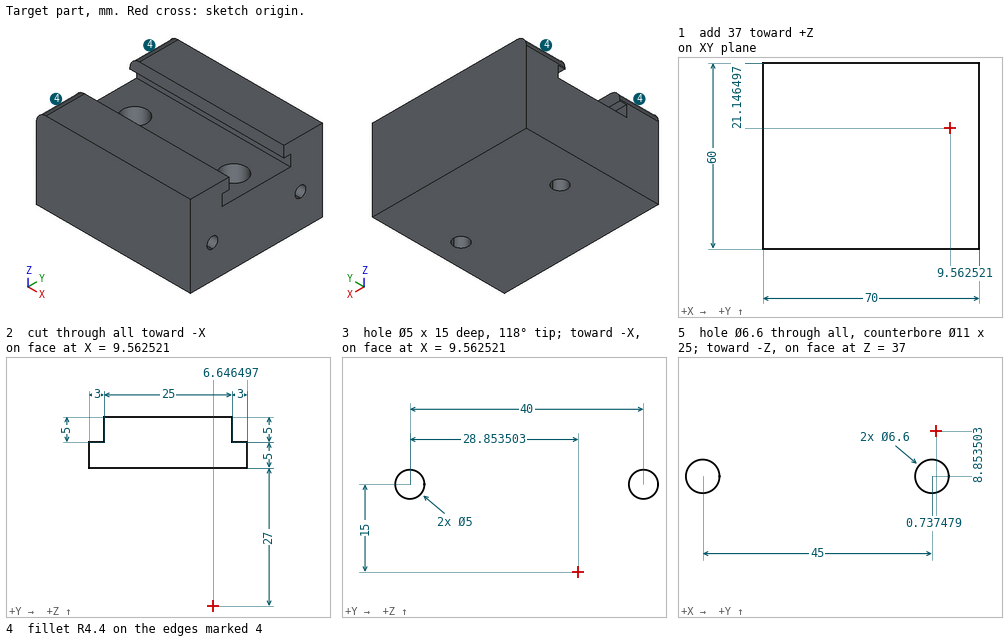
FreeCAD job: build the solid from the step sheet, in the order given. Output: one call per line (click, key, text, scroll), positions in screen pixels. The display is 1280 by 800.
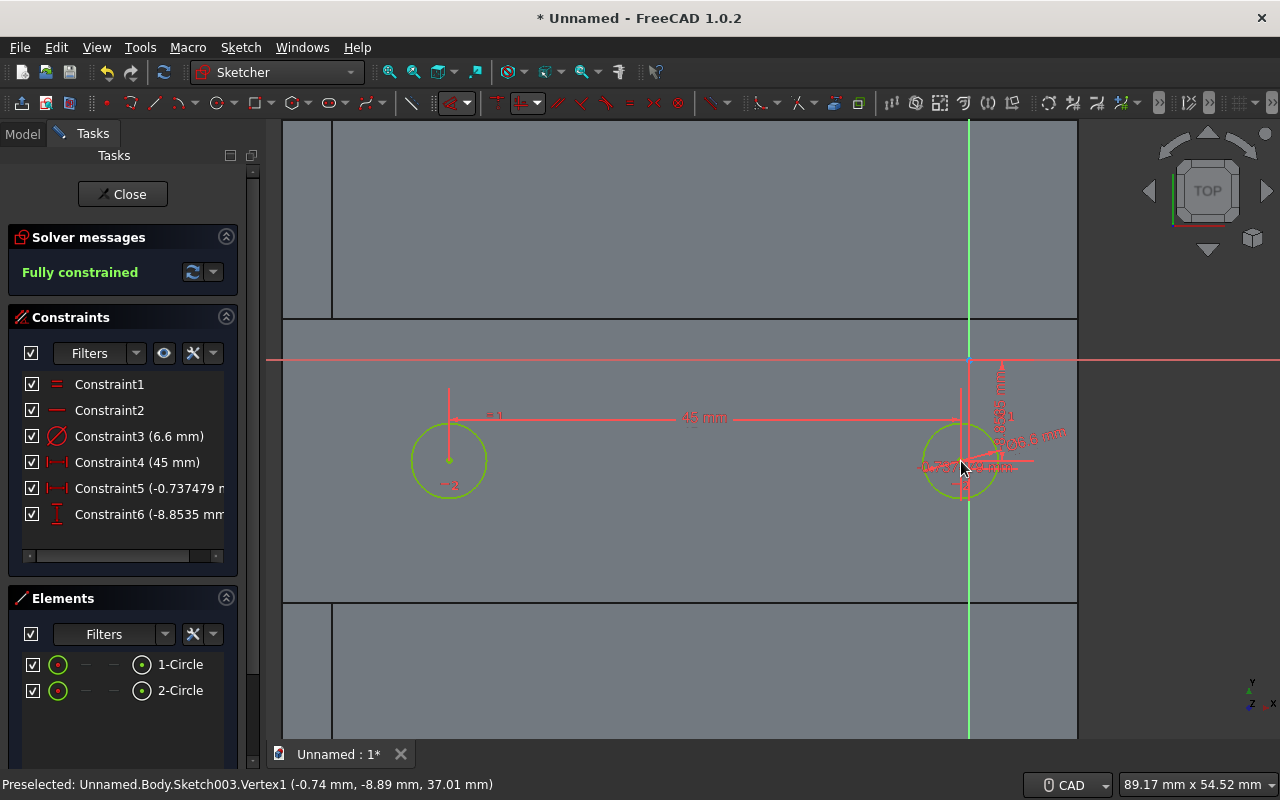
click(123, 194)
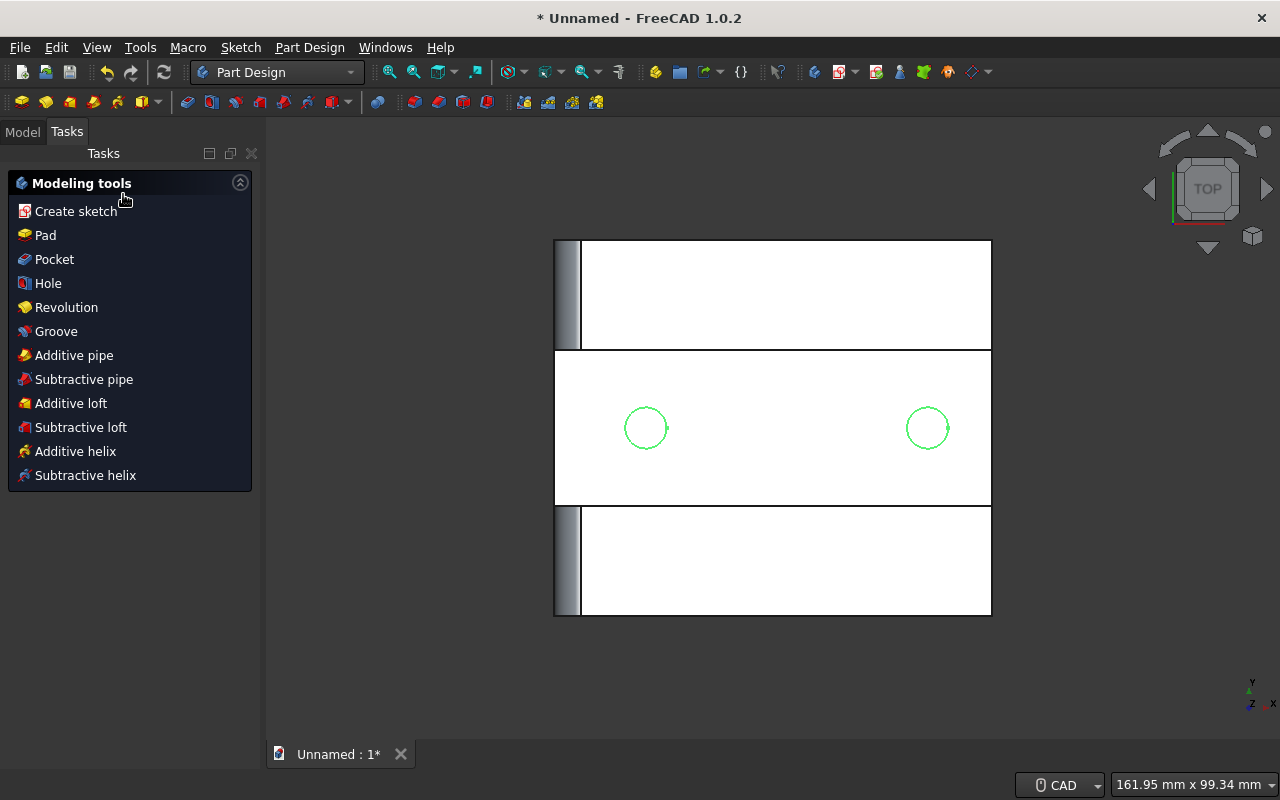
click(212, 102)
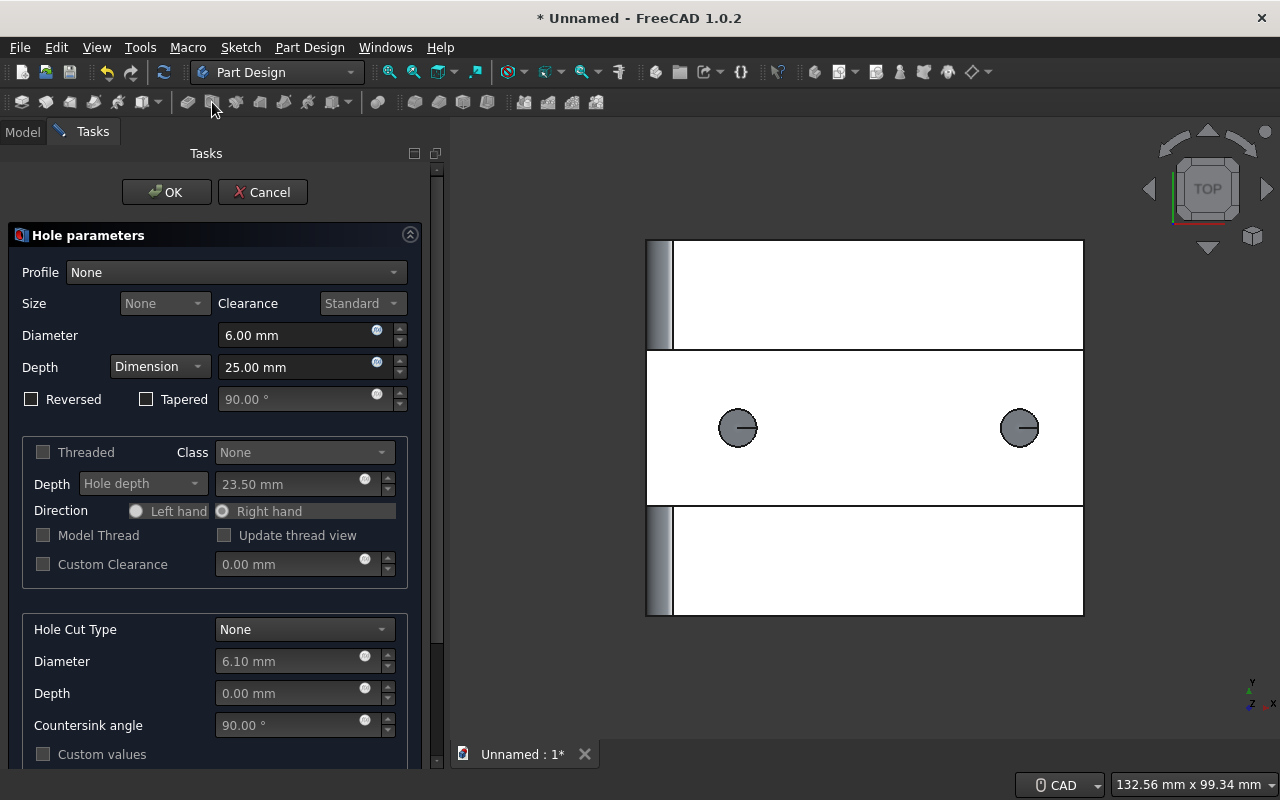
triple_click(305, 335)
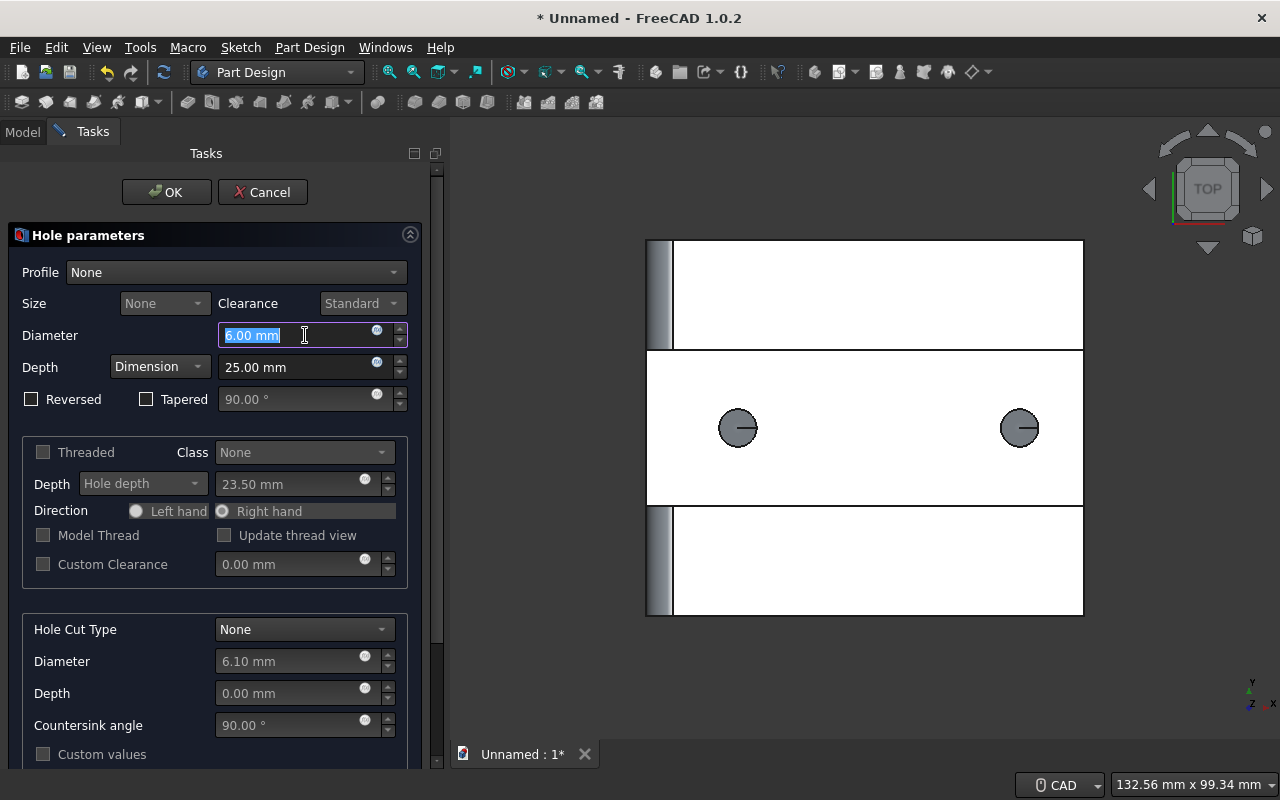
text(6.6)
key(Tab)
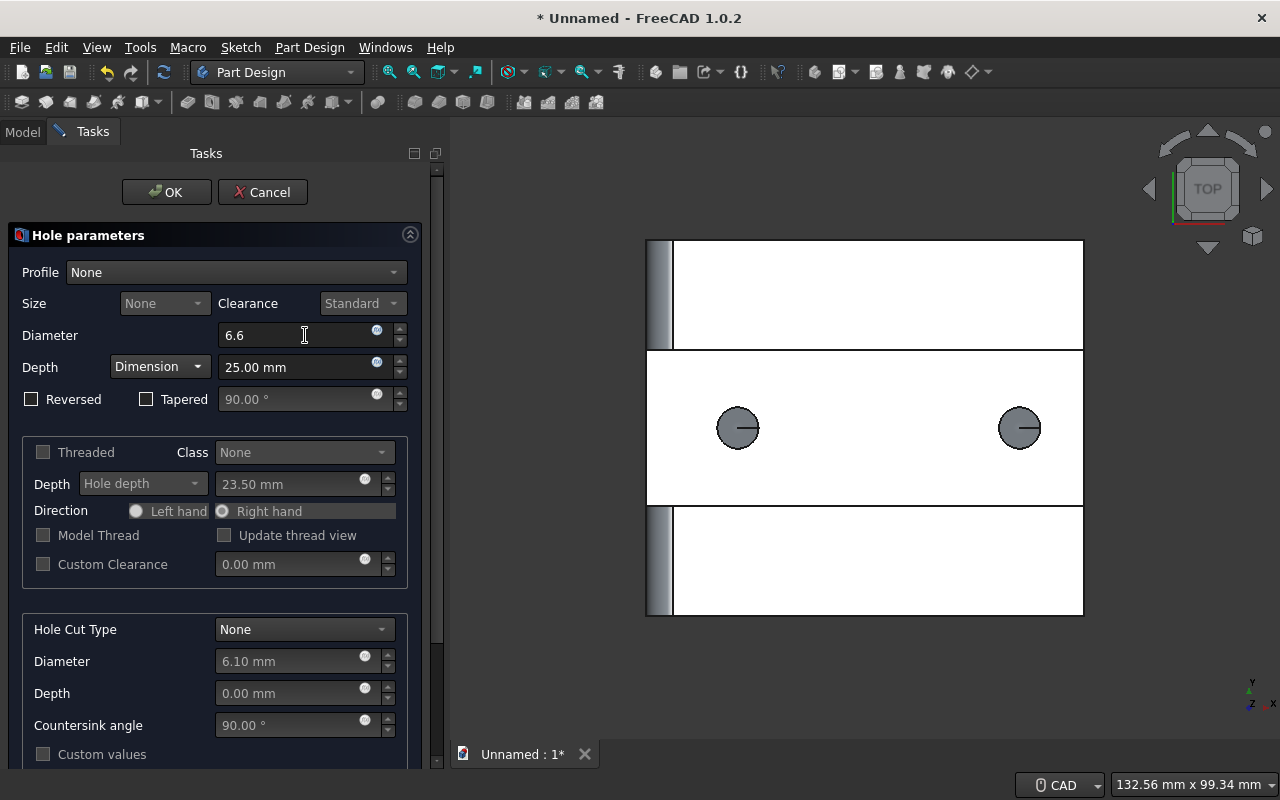
click(161, 366)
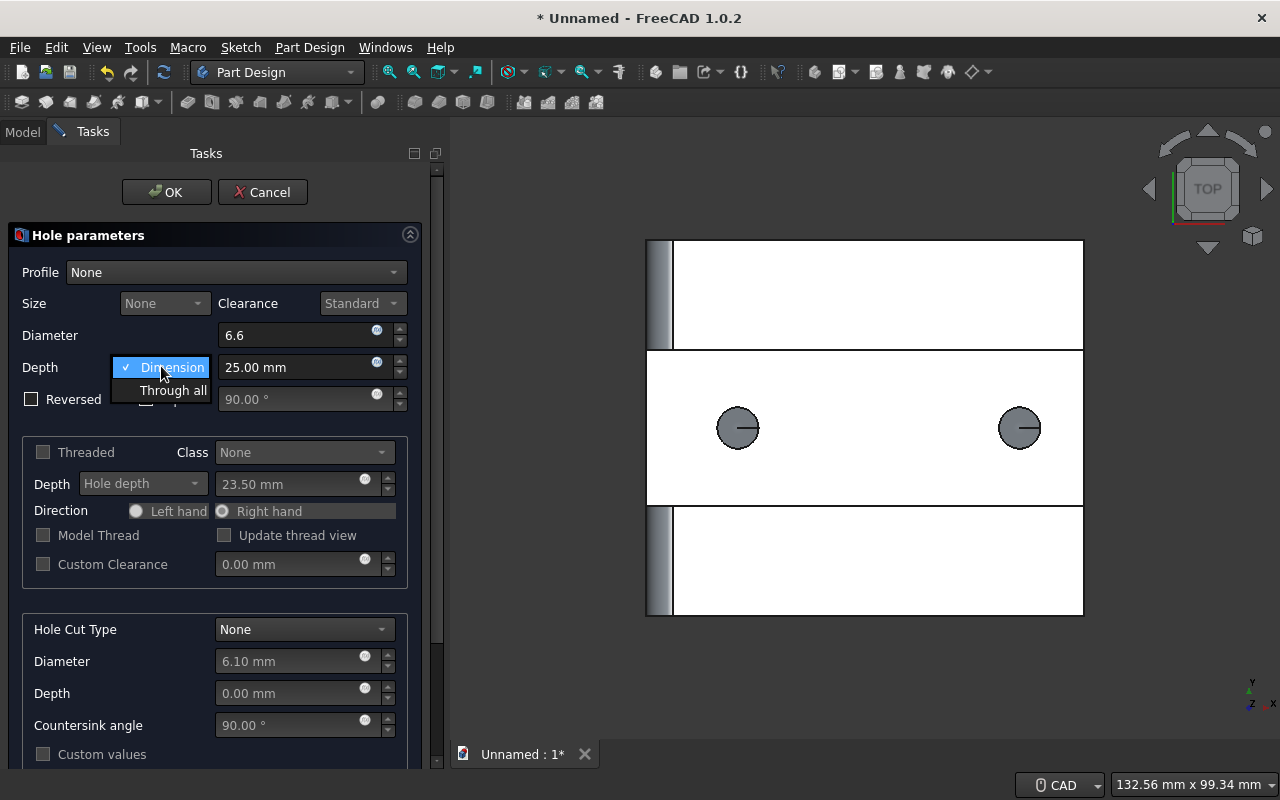
click(160, 390)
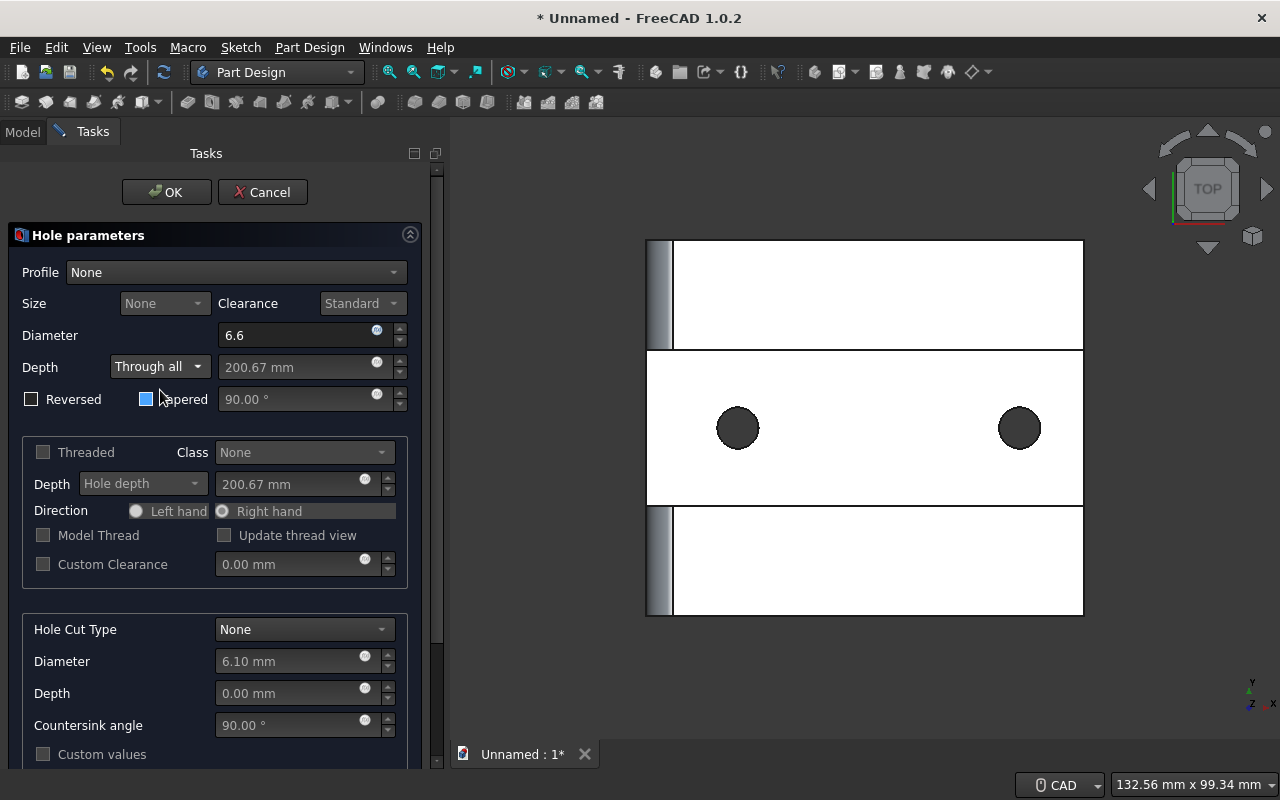
click(306, 630)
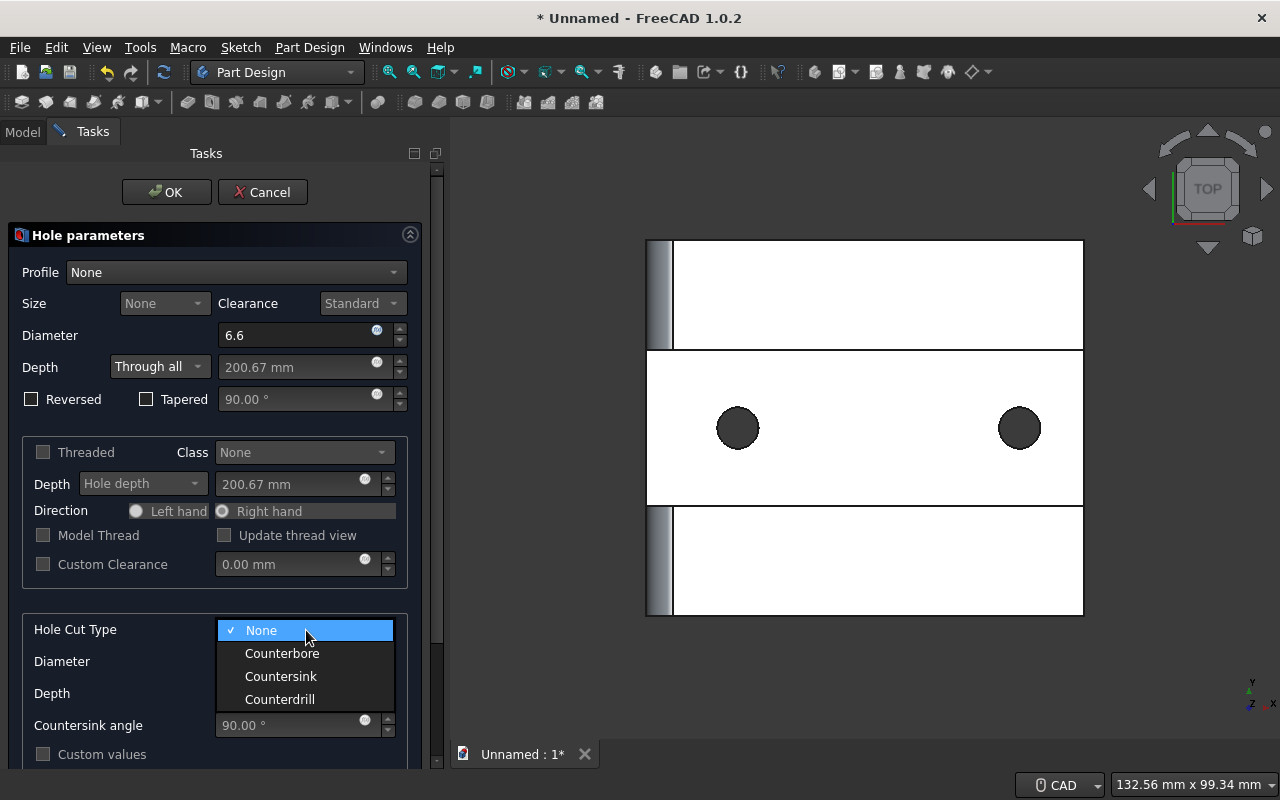
click(304, 654)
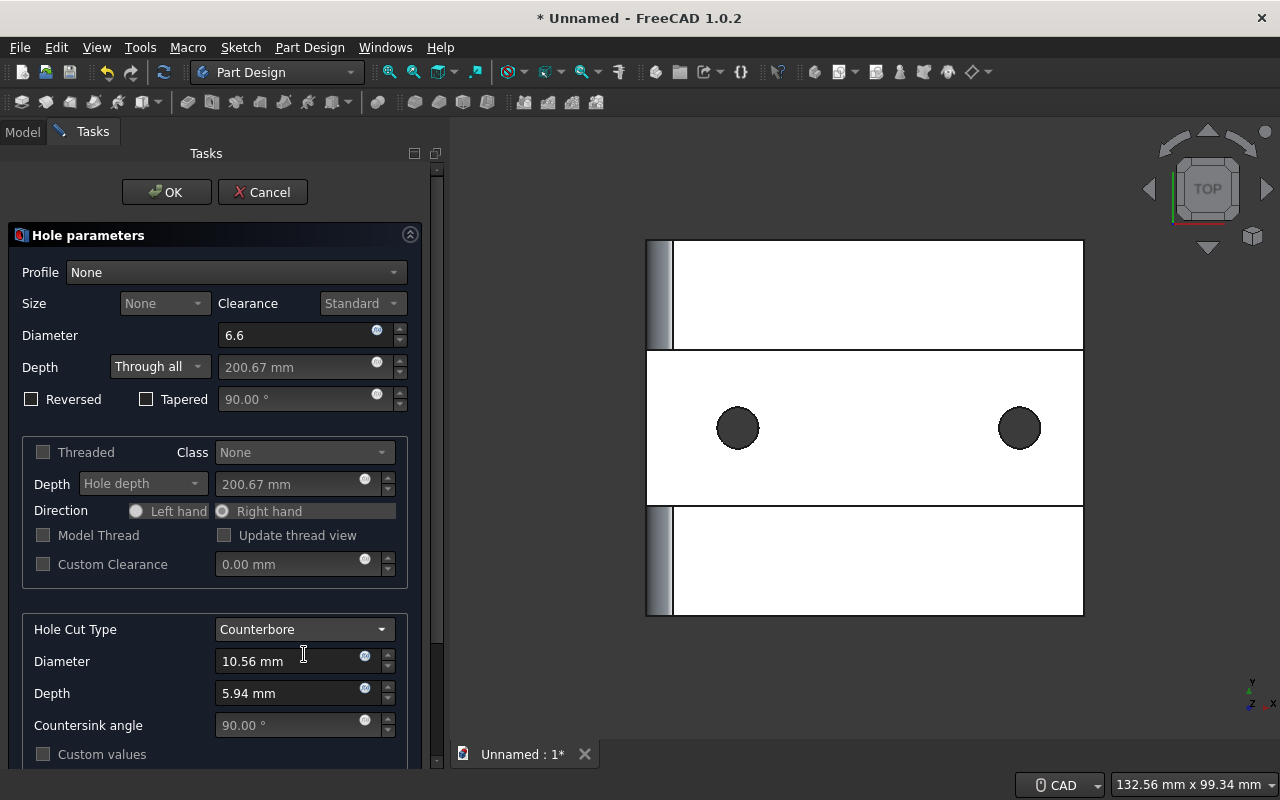
triple_click(298, 661)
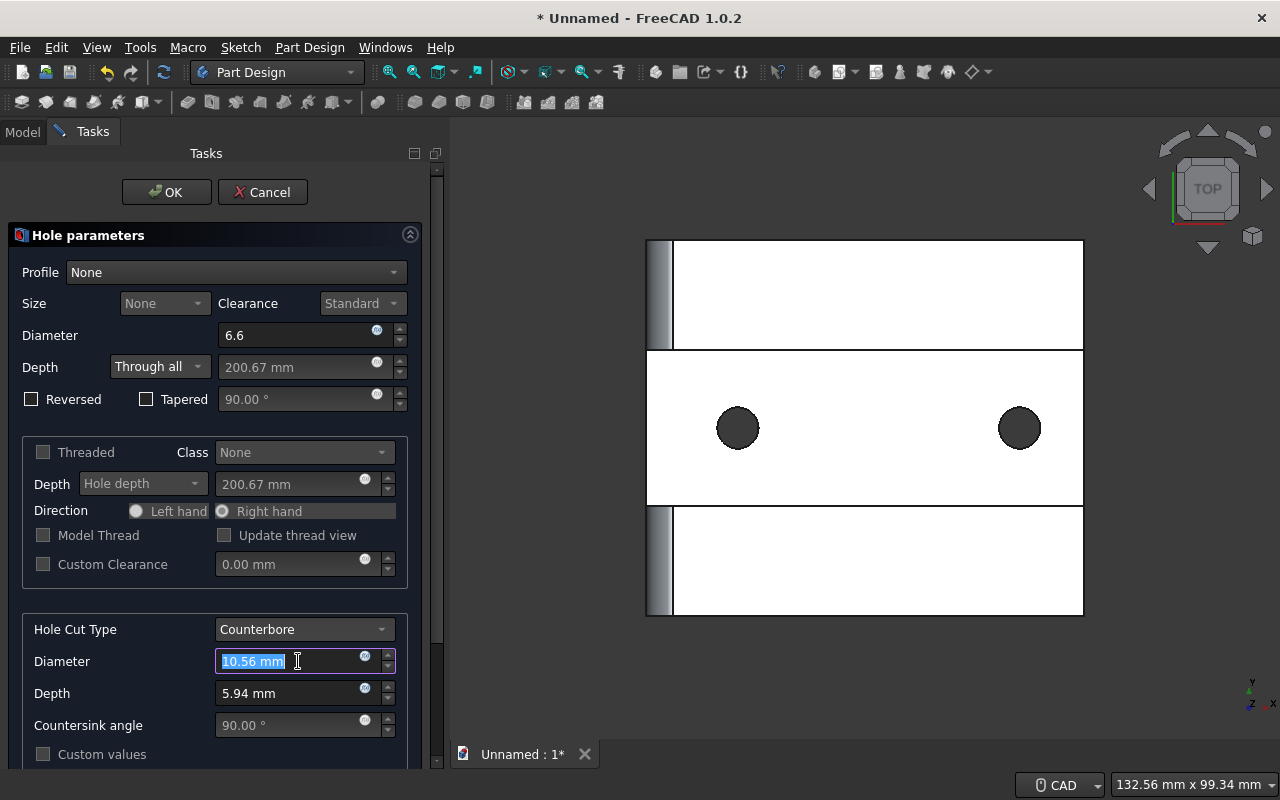
text(11)
key(Tab)